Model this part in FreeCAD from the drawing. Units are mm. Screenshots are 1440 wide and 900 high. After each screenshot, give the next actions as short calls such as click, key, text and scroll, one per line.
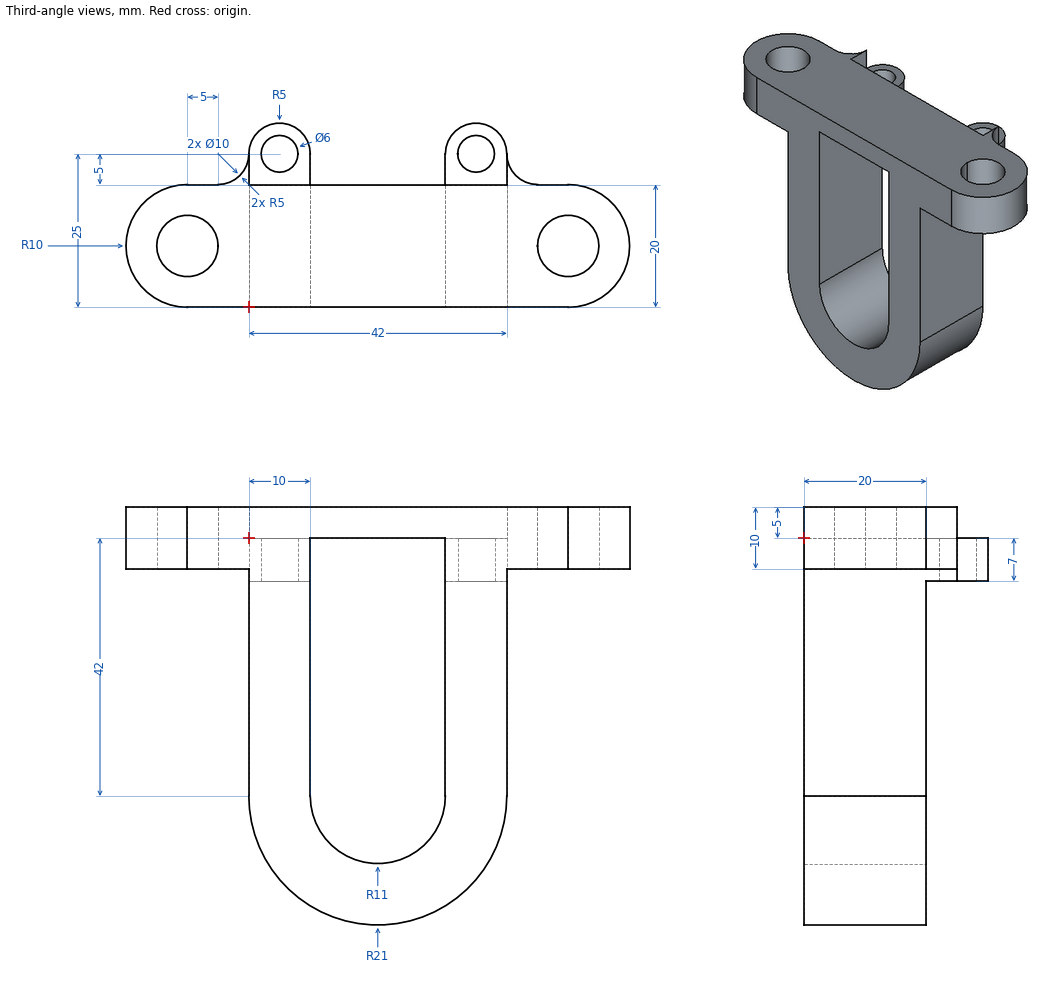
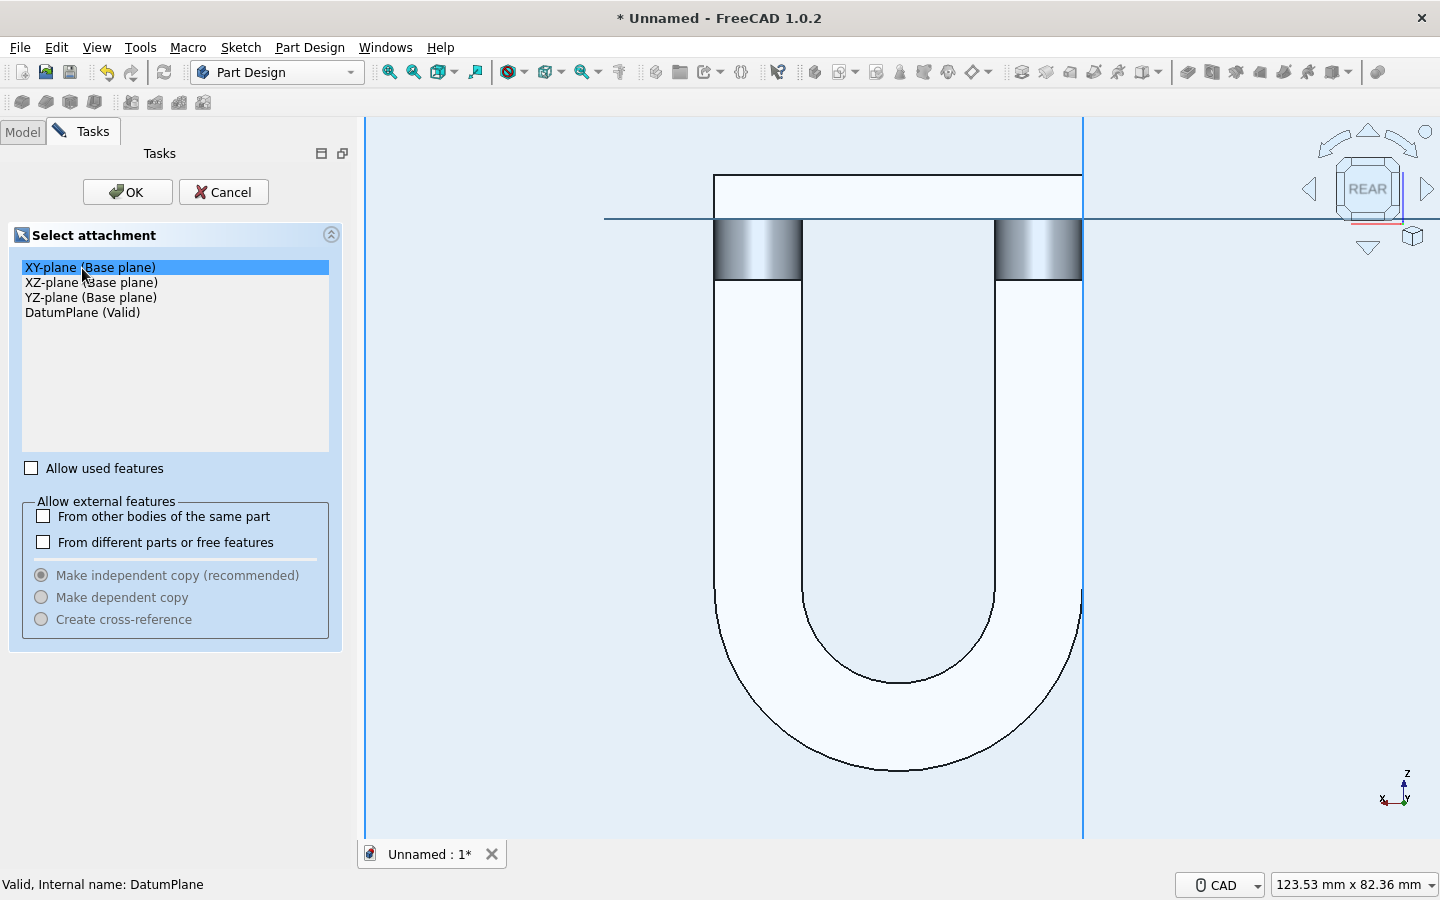
click(128, 192)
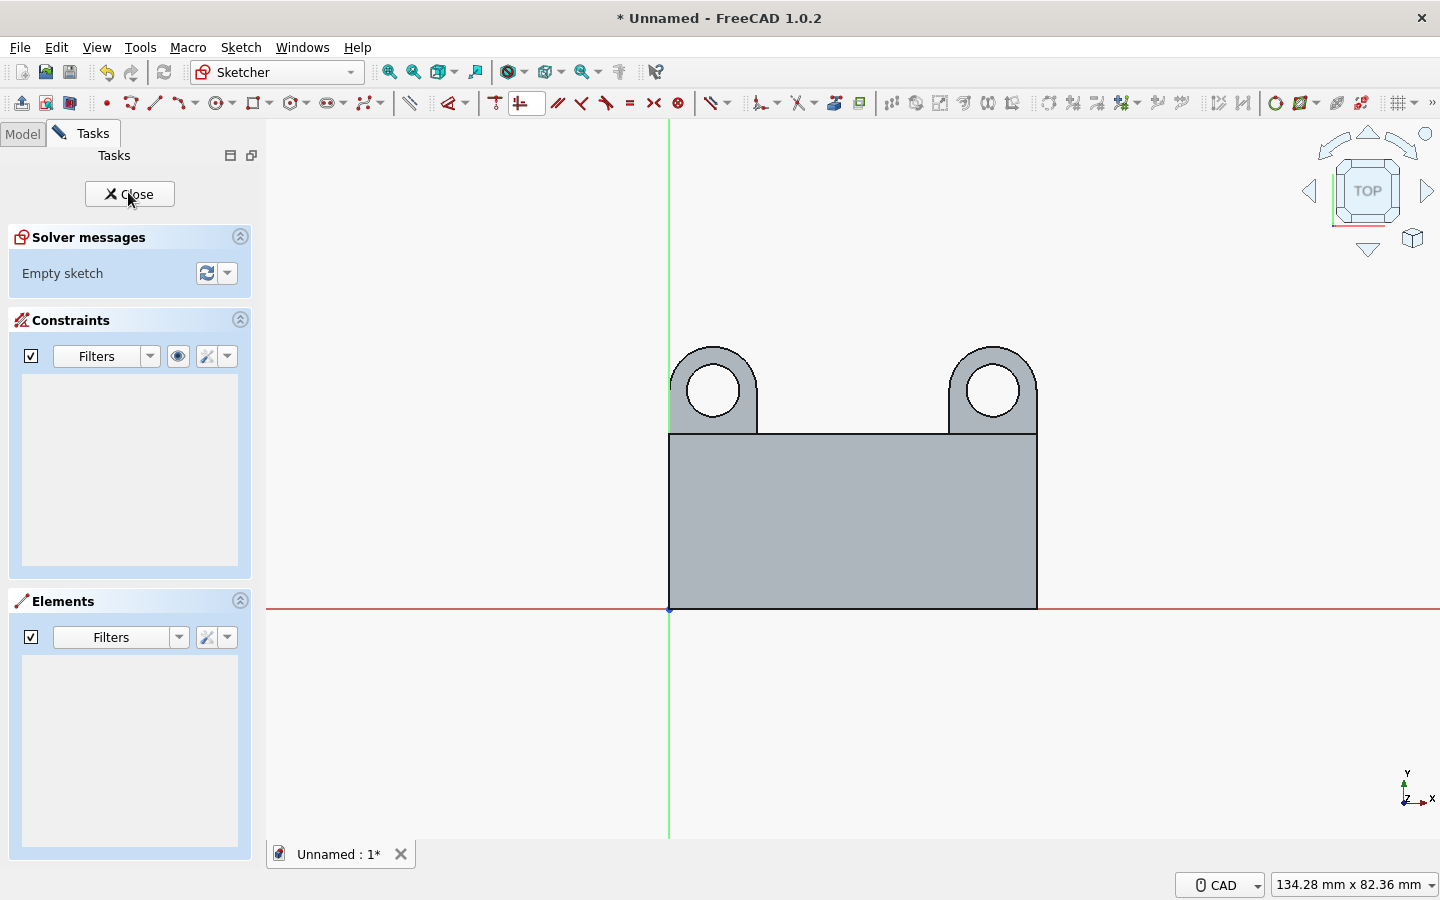
click(70, 104)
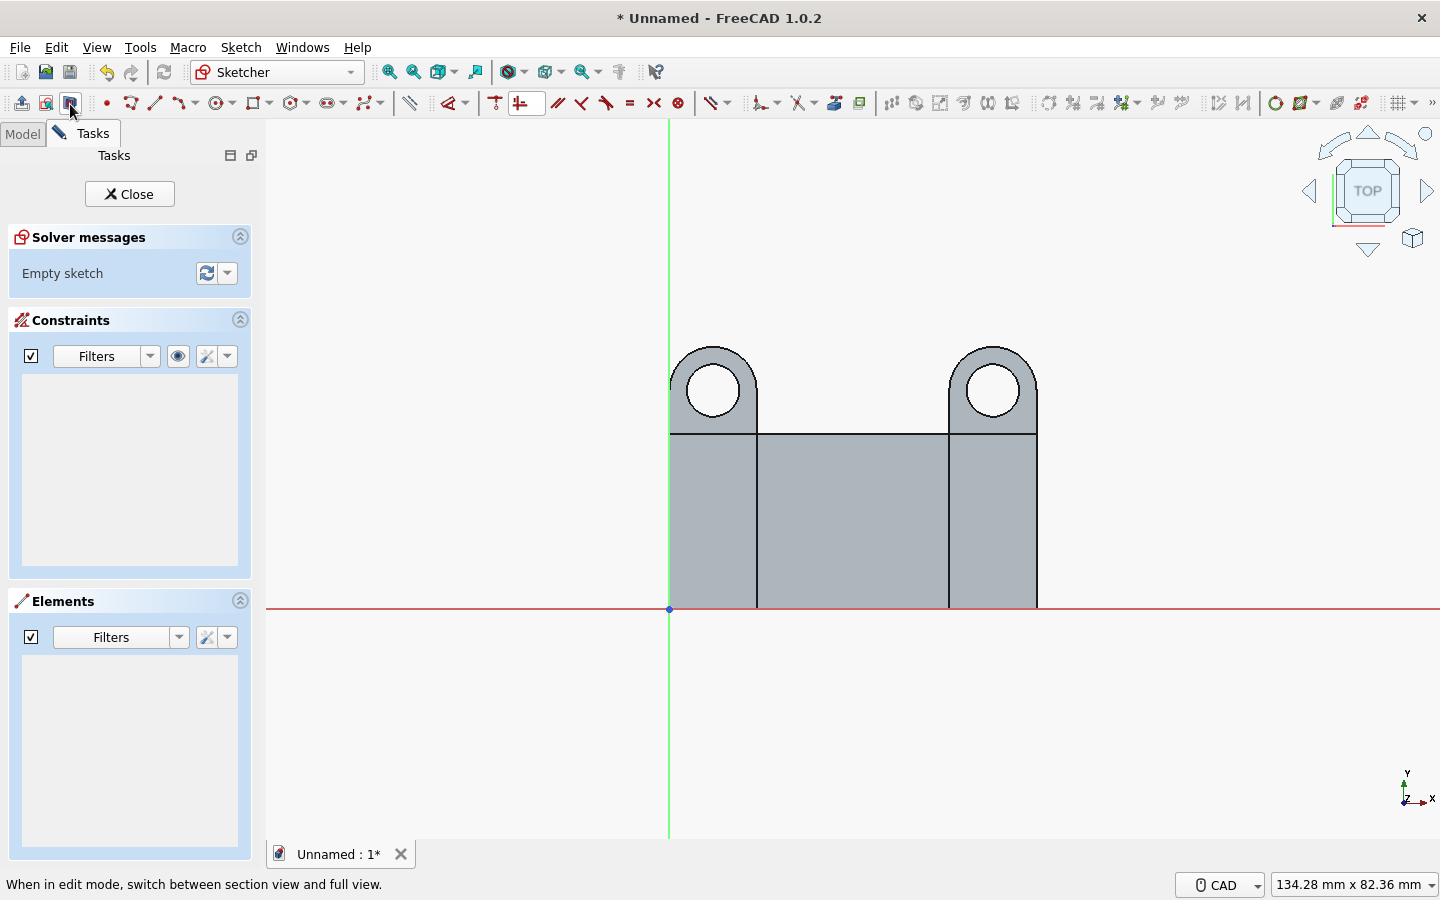
scroll(417, 517, up, 4)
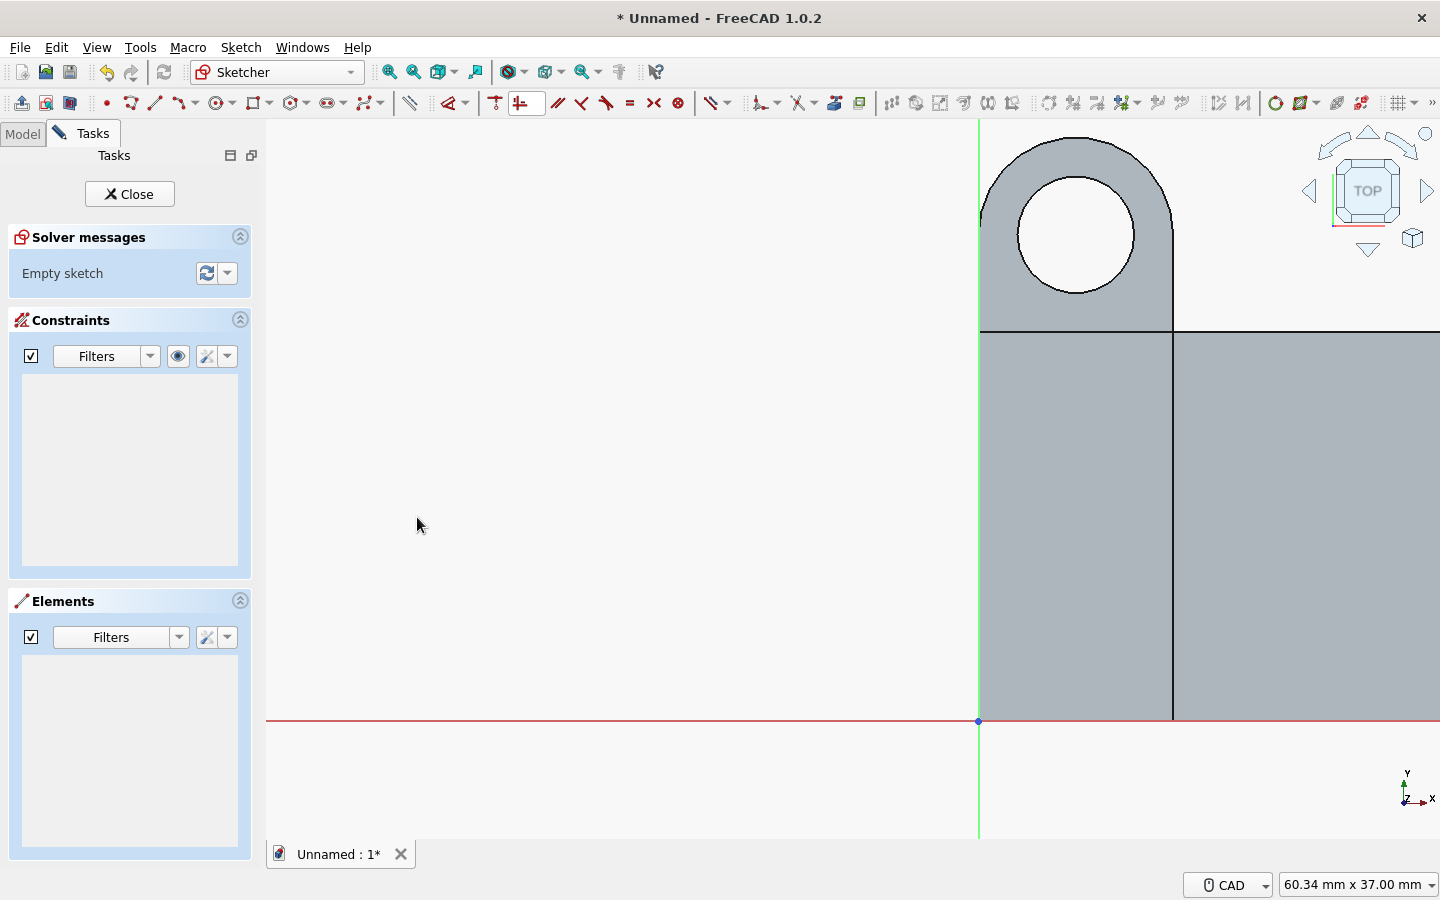
click(156, 104)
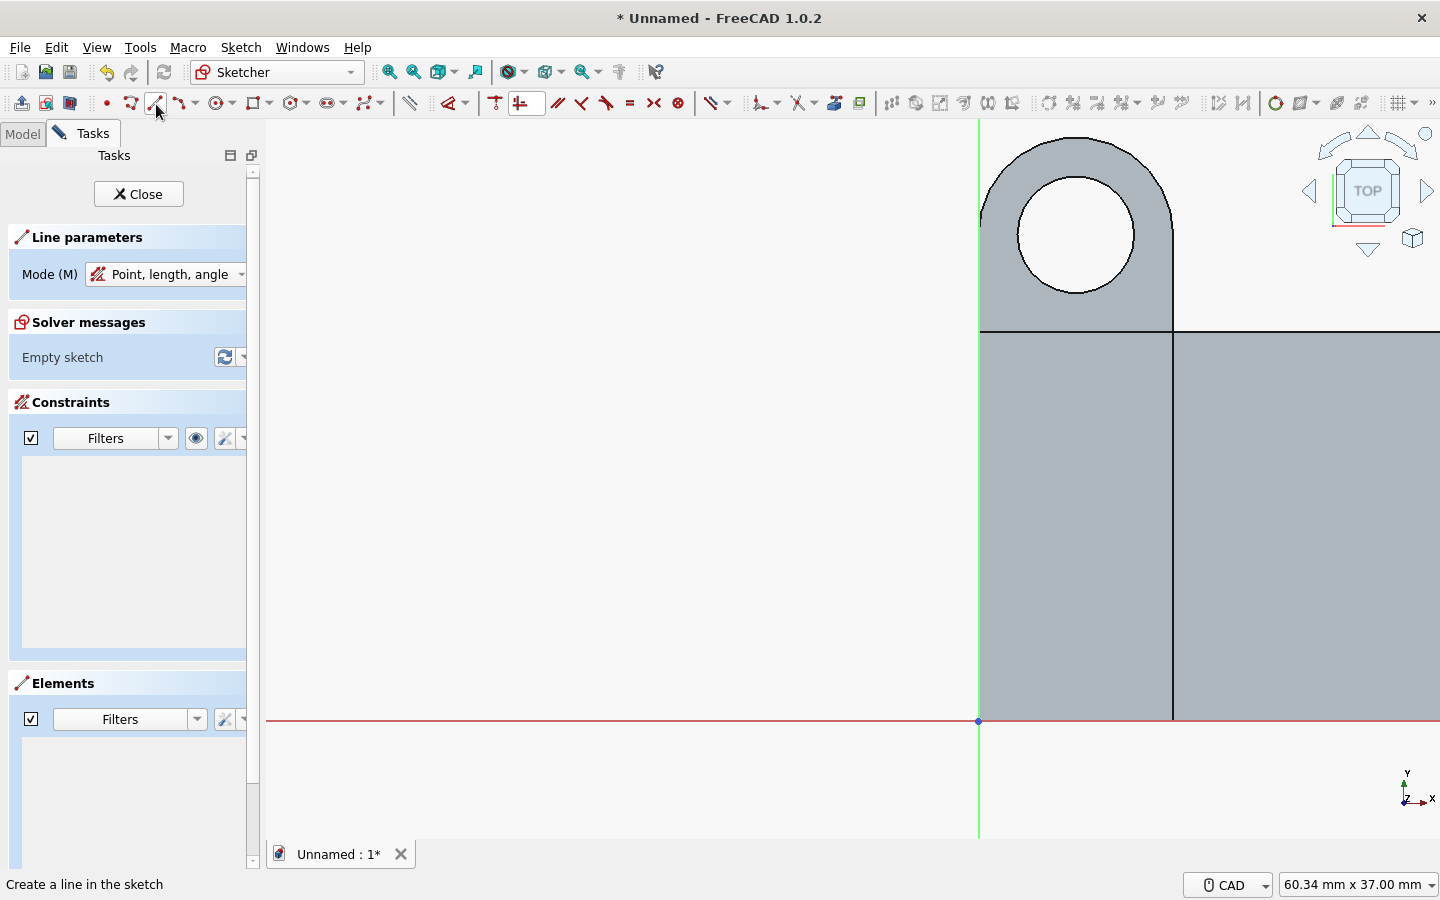
click(881, 332)
click(784, 332)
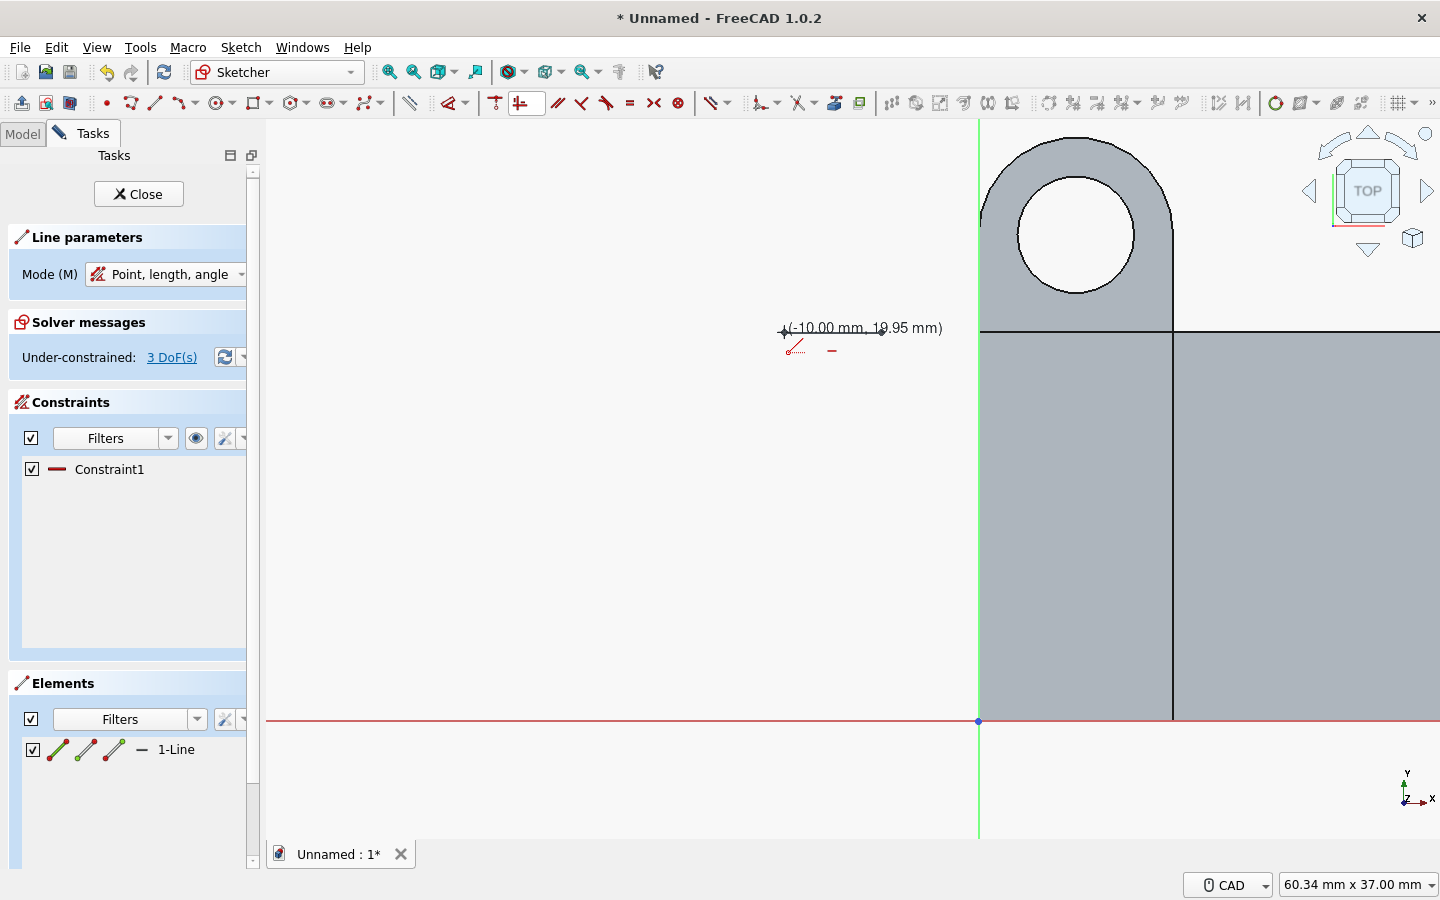
click(132, 104)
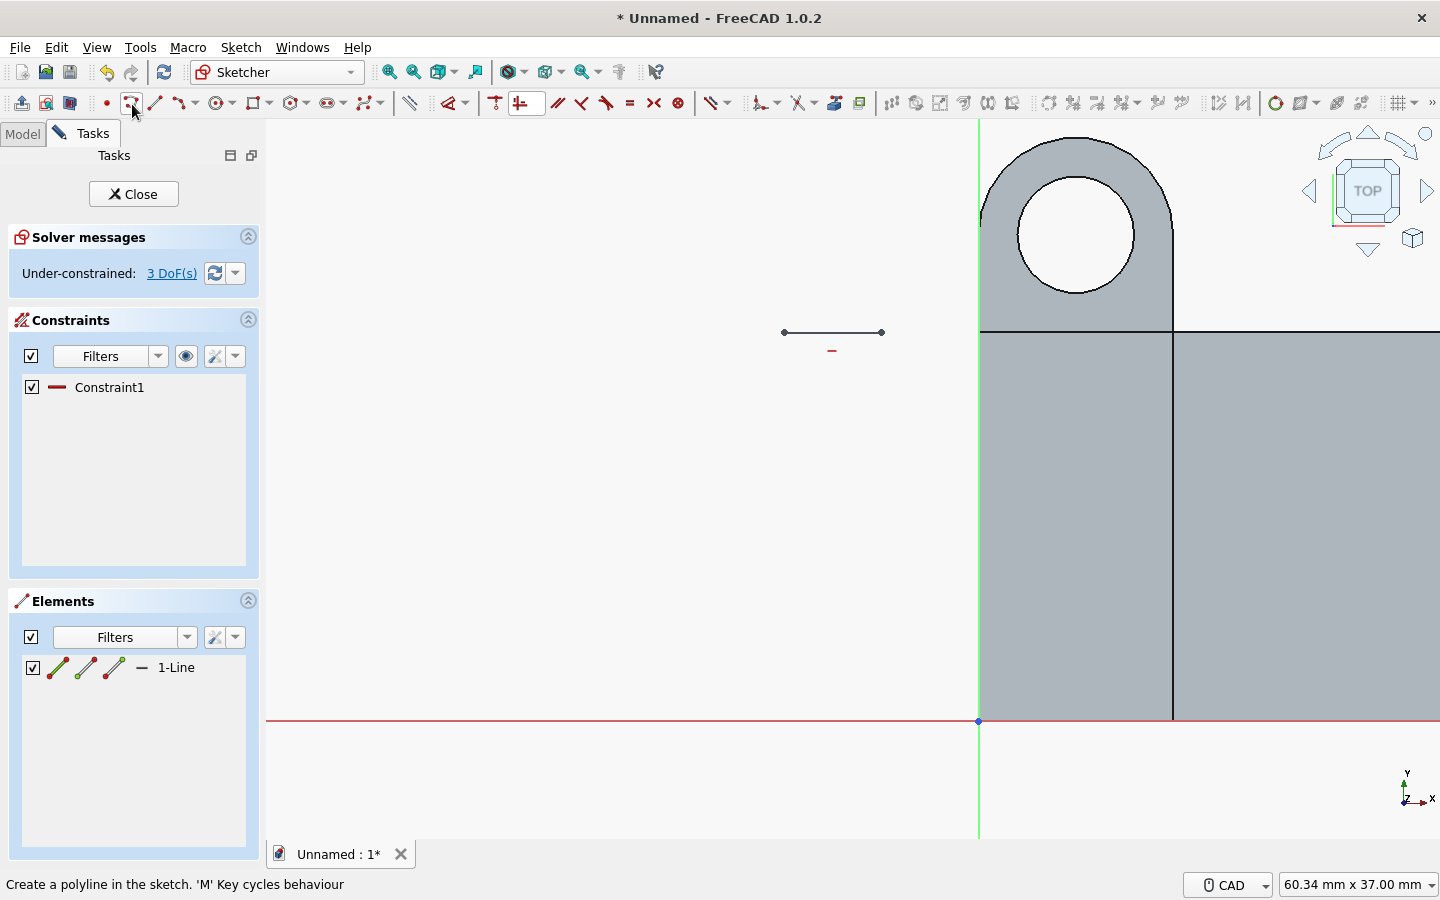
click(784, 721)
click(979, 721)
click(970, 235)
right_click(970, 235)